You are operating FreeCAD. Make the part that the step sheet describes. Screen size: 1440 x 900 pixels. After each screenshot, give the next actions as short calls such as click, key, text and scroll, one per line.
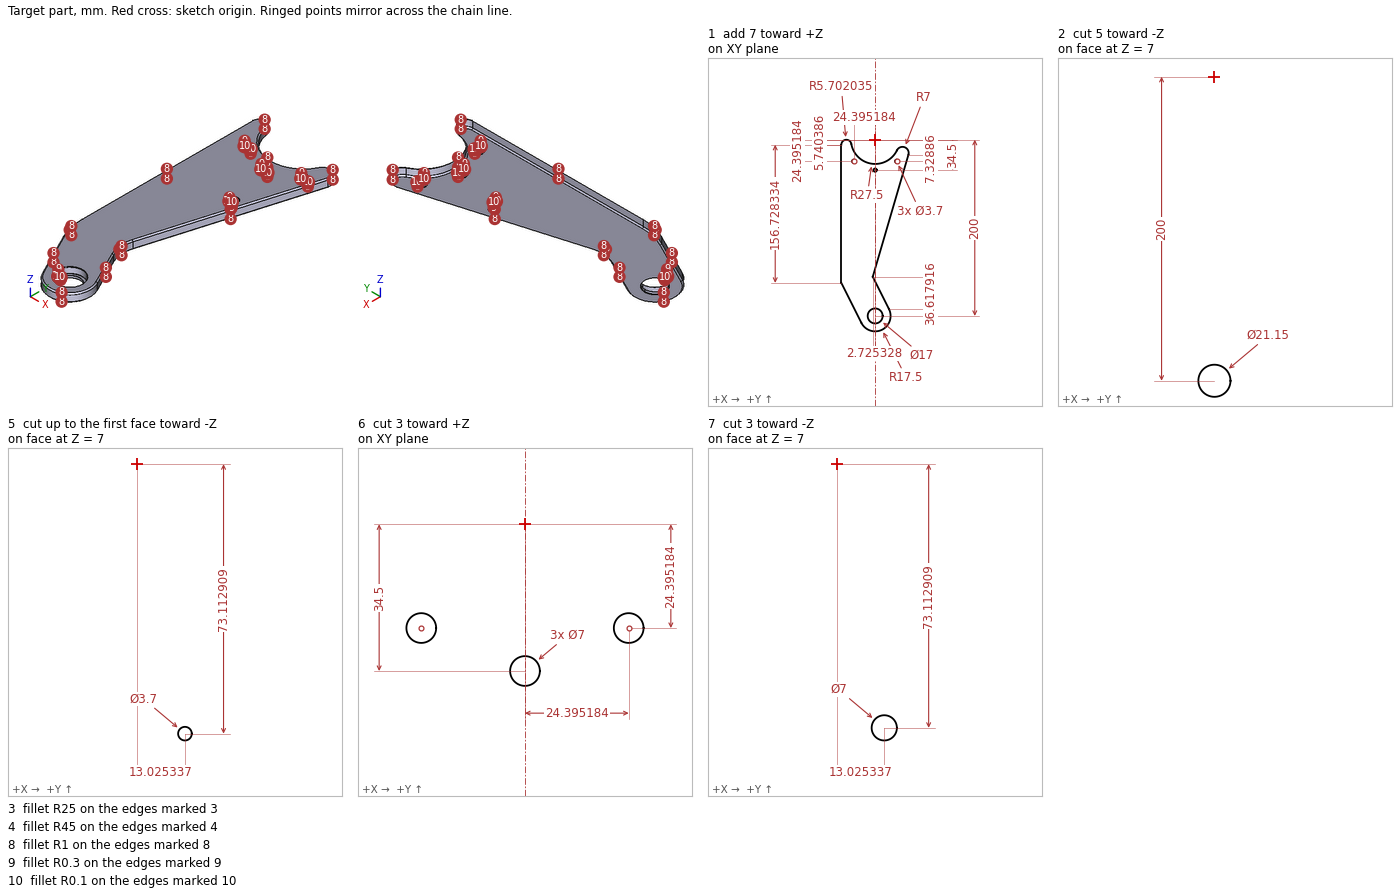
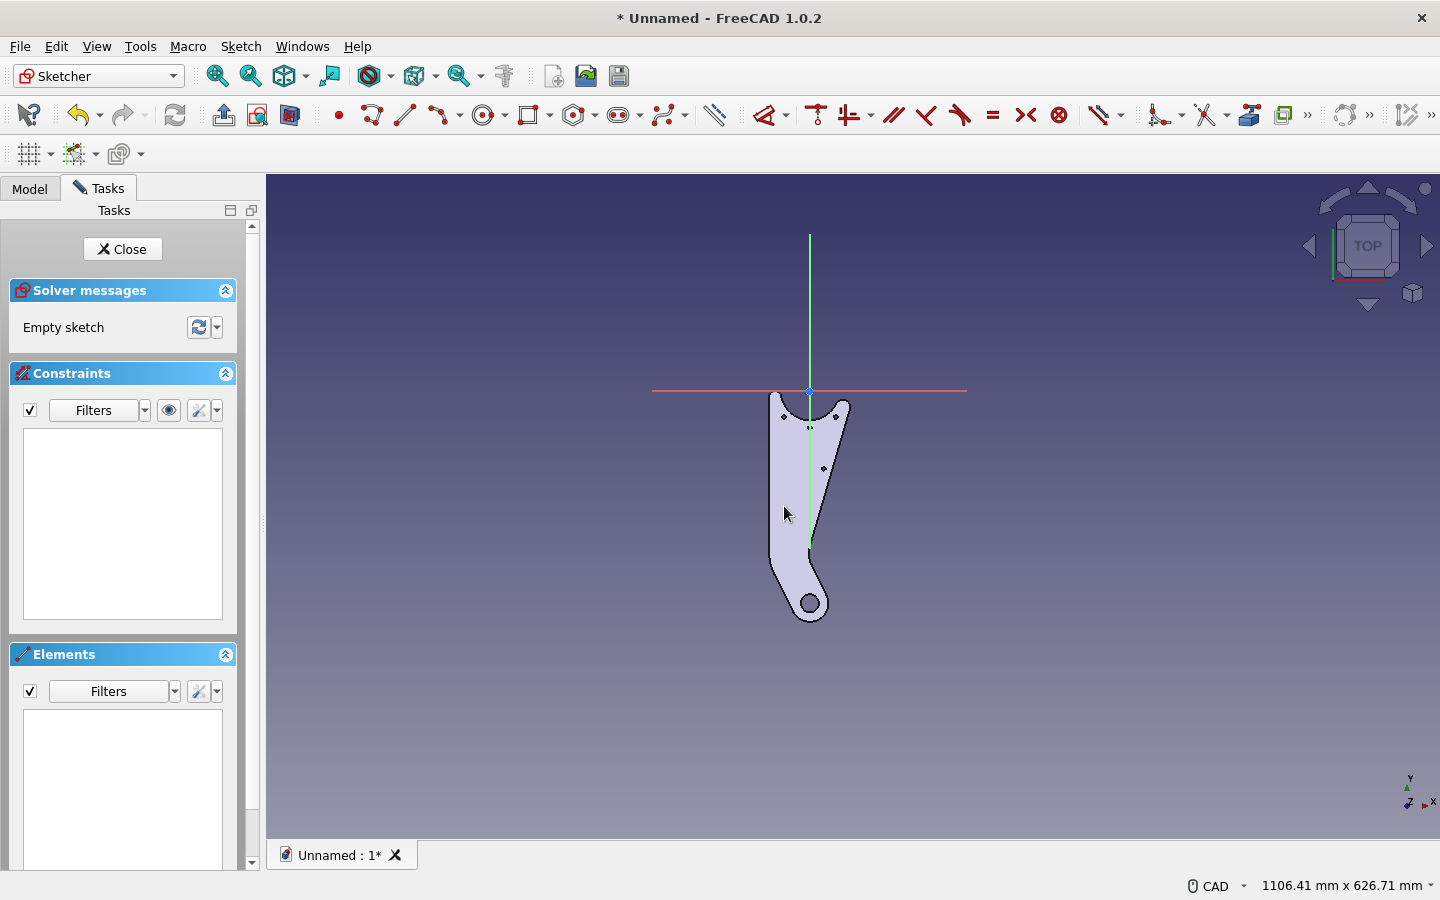
scroll(812, 402, up, 12)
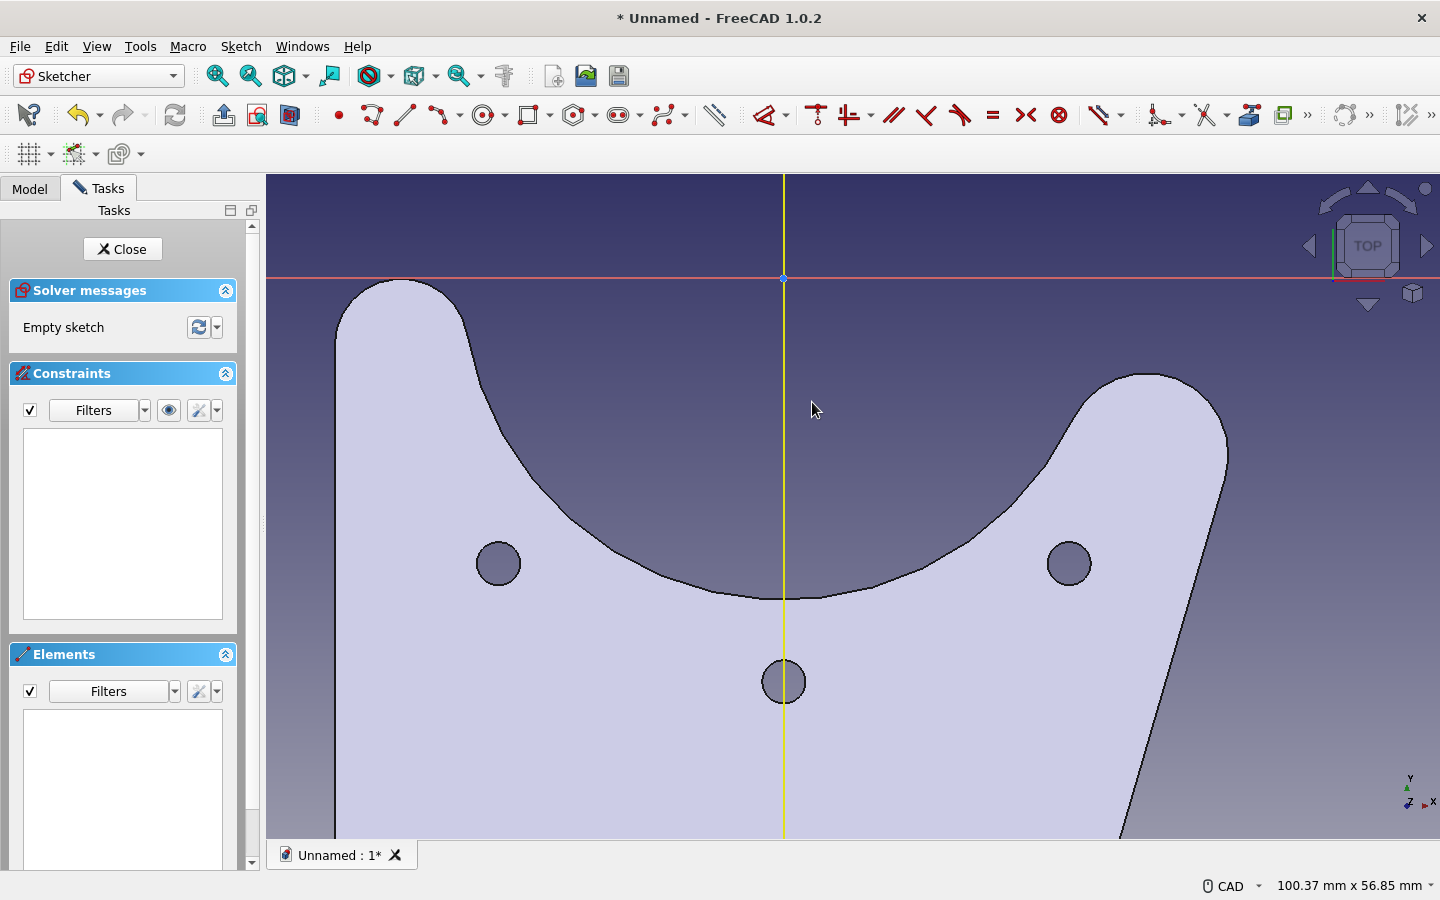
click(482, 116)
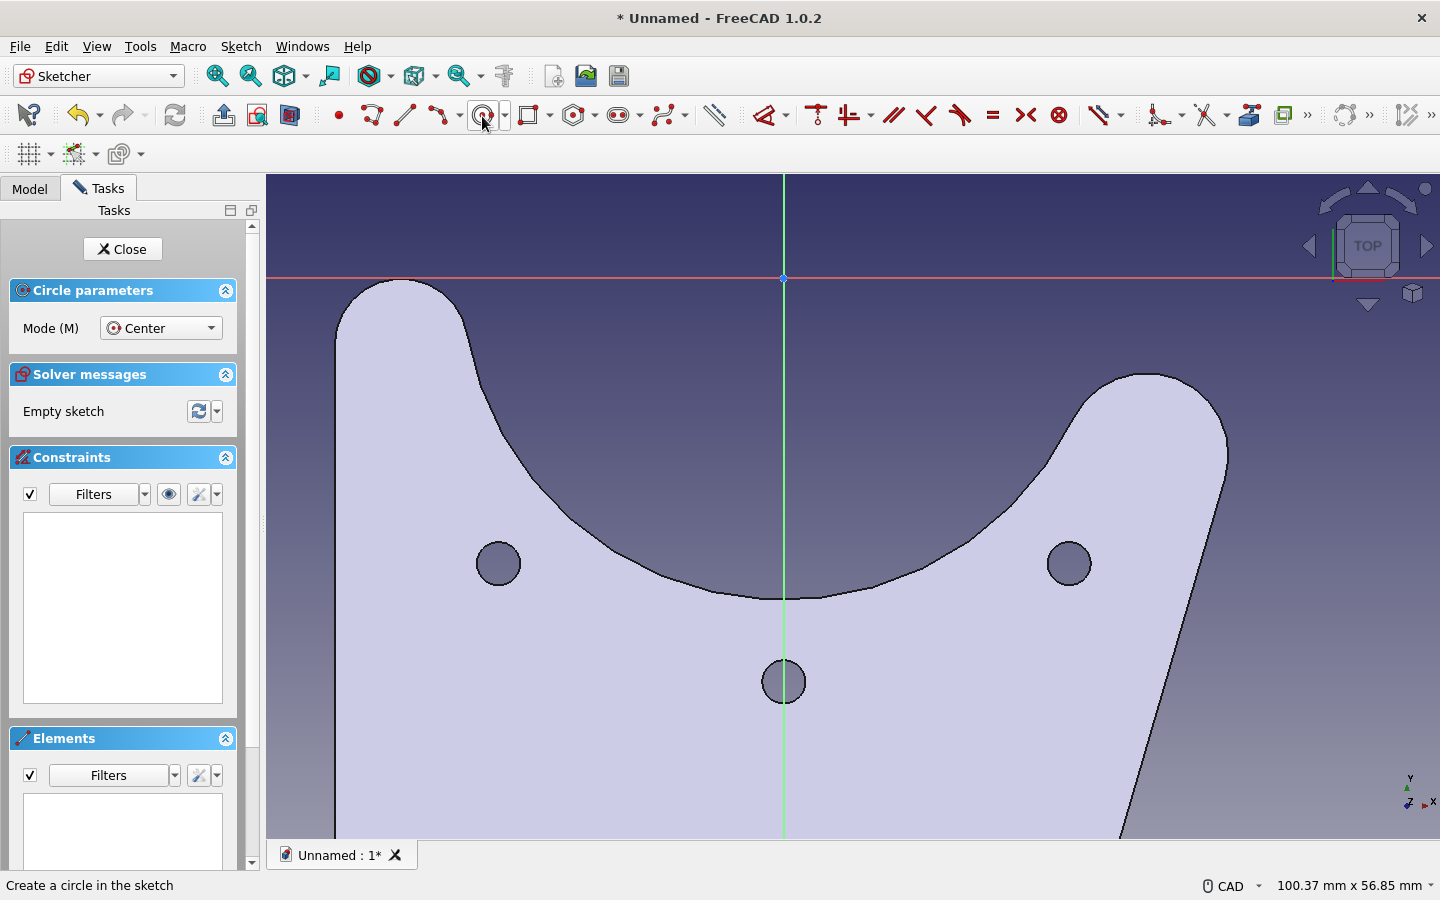
click(784, 682)
click(813, 653)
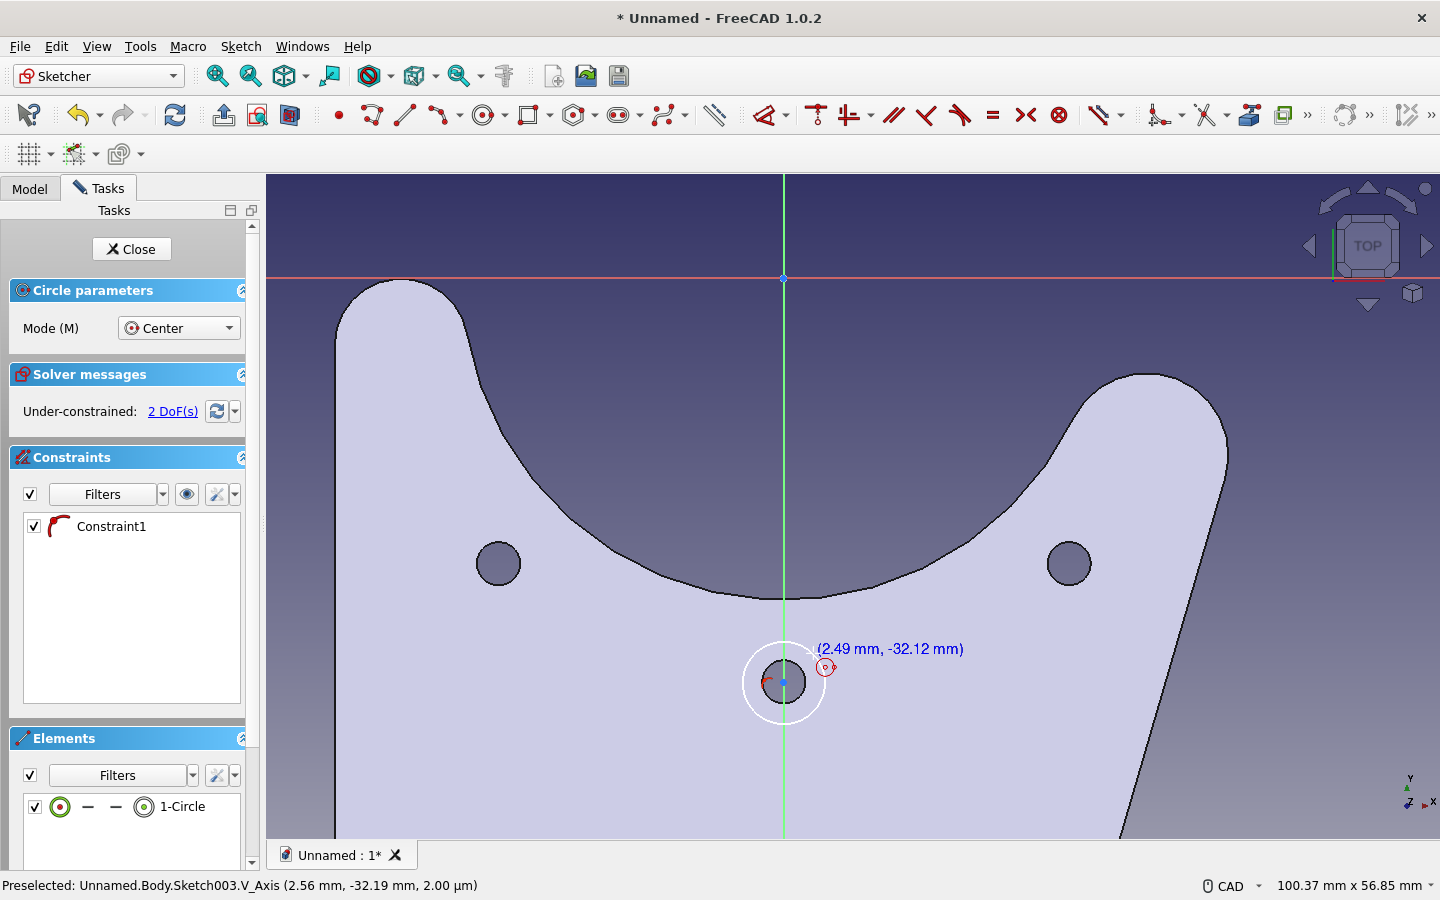
click(1069, 564)
click(1098, 535)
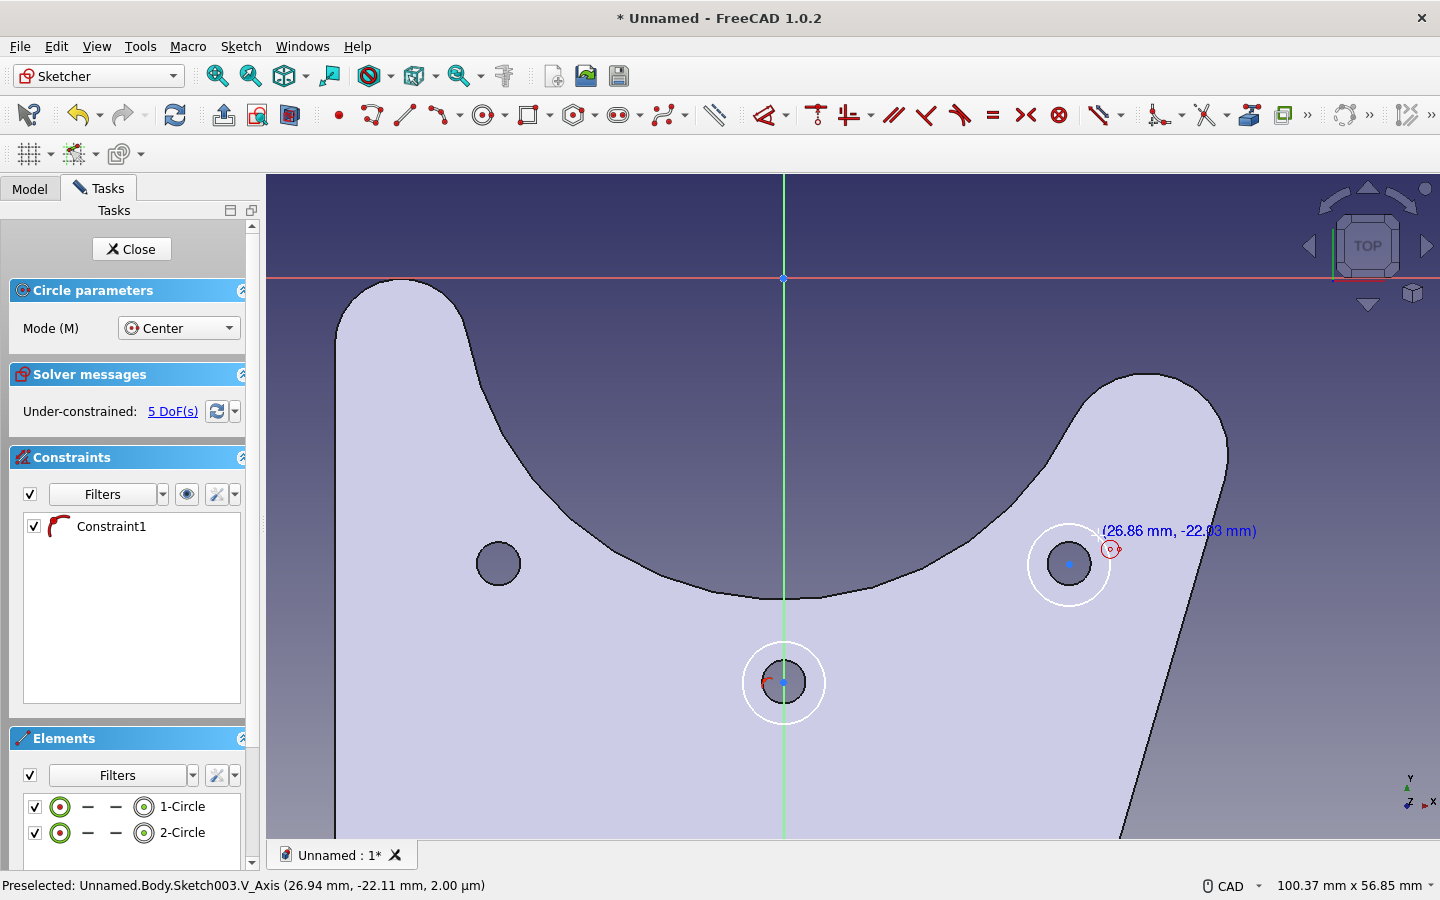
click(499, 564)
click(527, 535)
key(Escape)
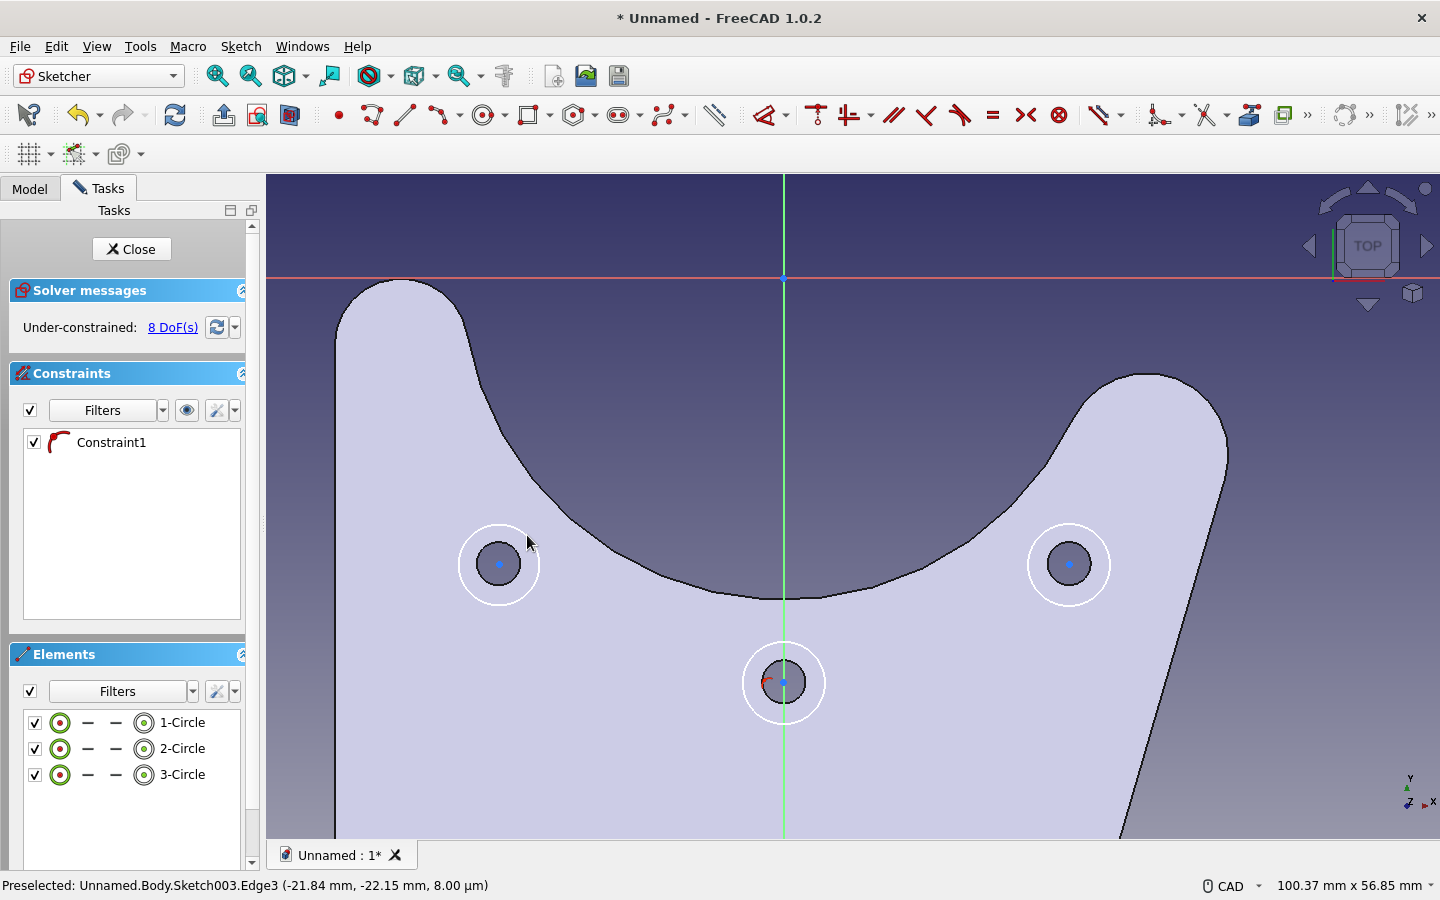
click(813, 654)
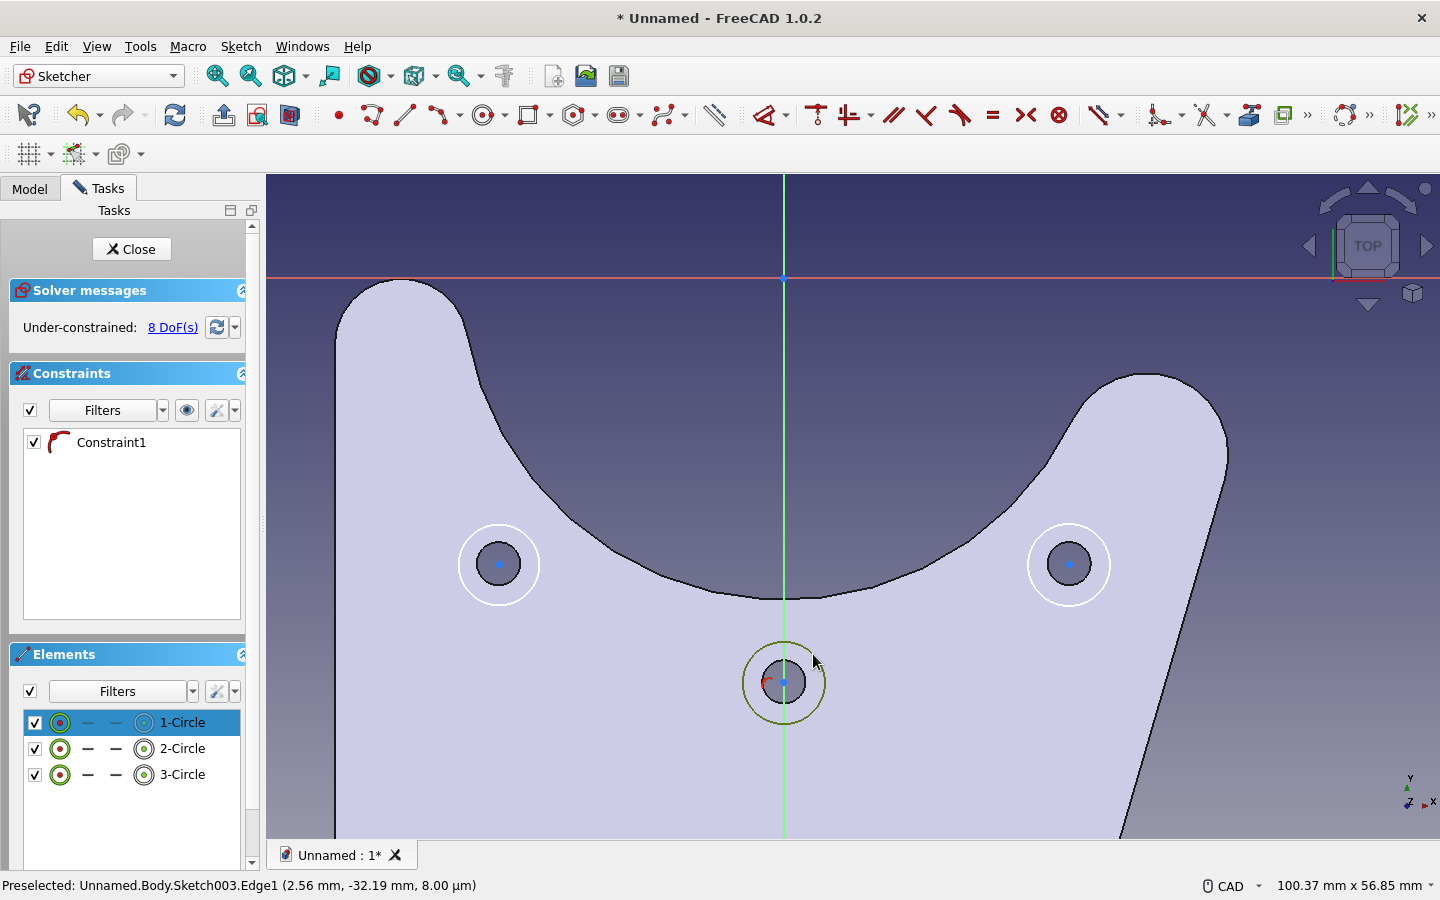
click(1098, 536)